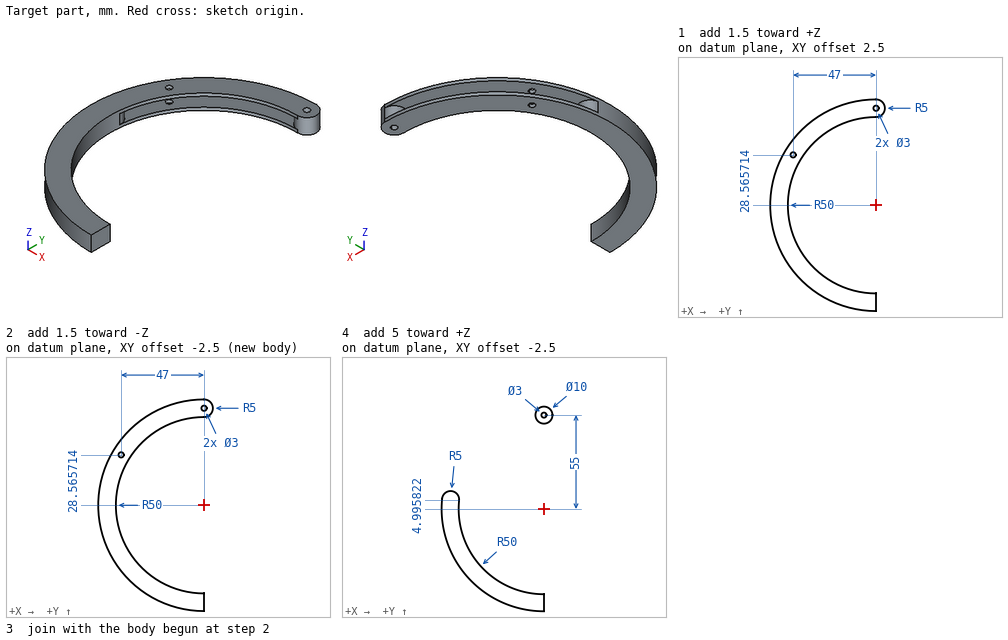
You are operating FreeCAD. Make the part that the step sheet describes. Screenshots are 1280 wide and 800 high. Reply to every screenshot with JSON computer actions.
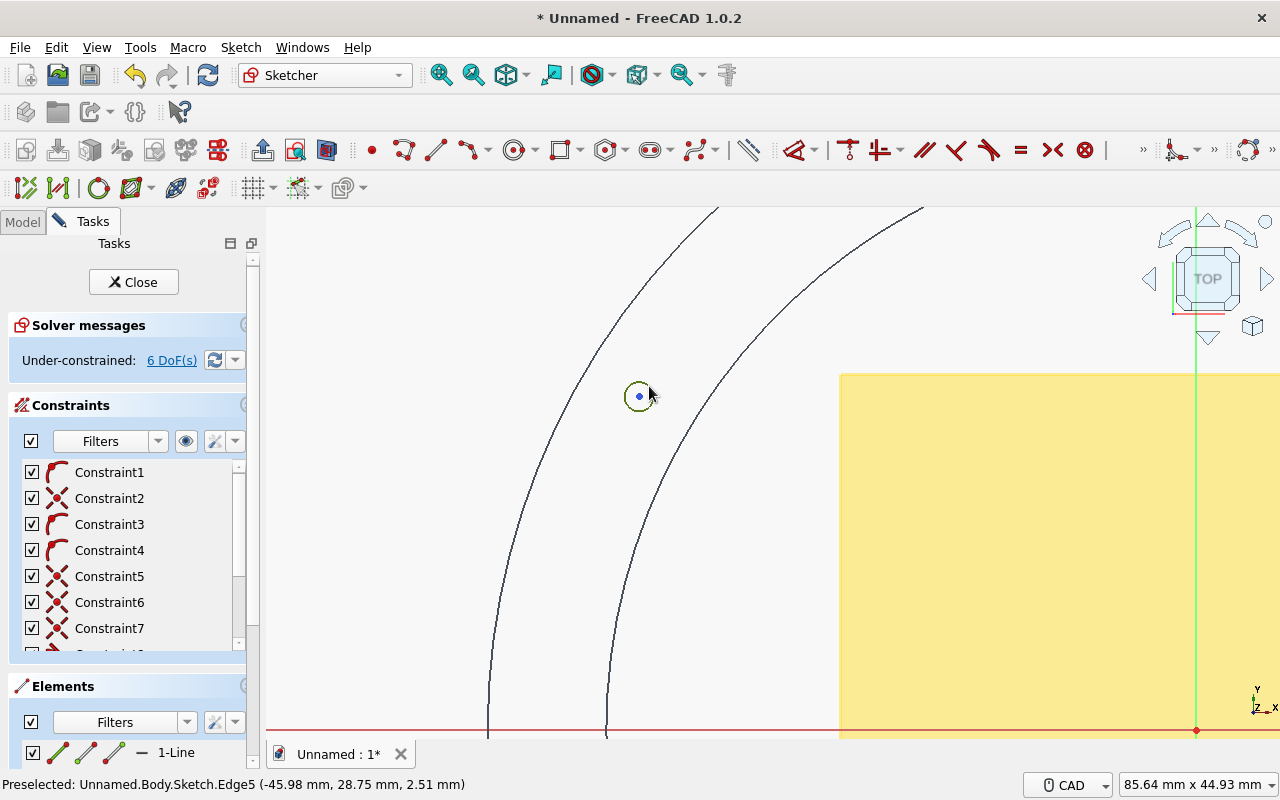
{"action": "scroll", "coordinate": [650, 389], "scroll_direction": "down", "scroll_amount": 7}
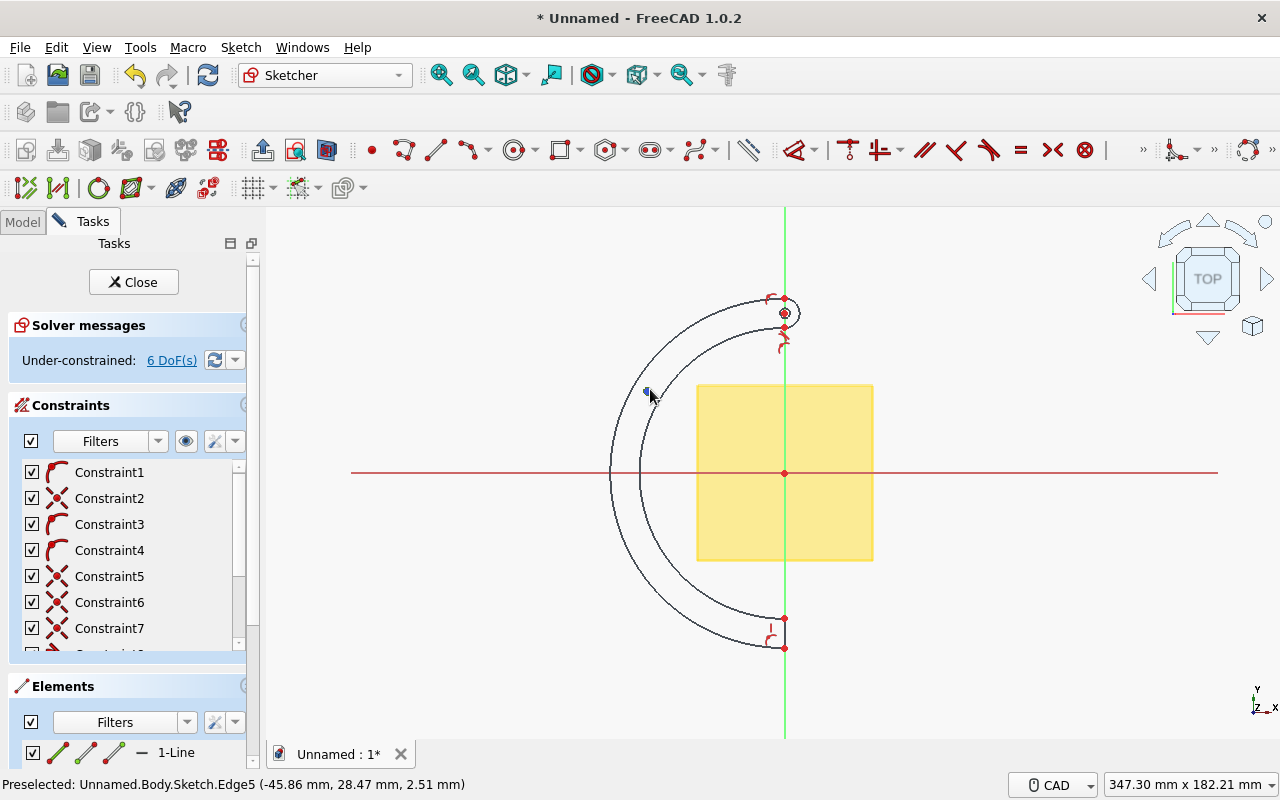
{"action": "scroll", "coordinate": [788, 310], "scroll_direction": "up", "scroll_amount": 7}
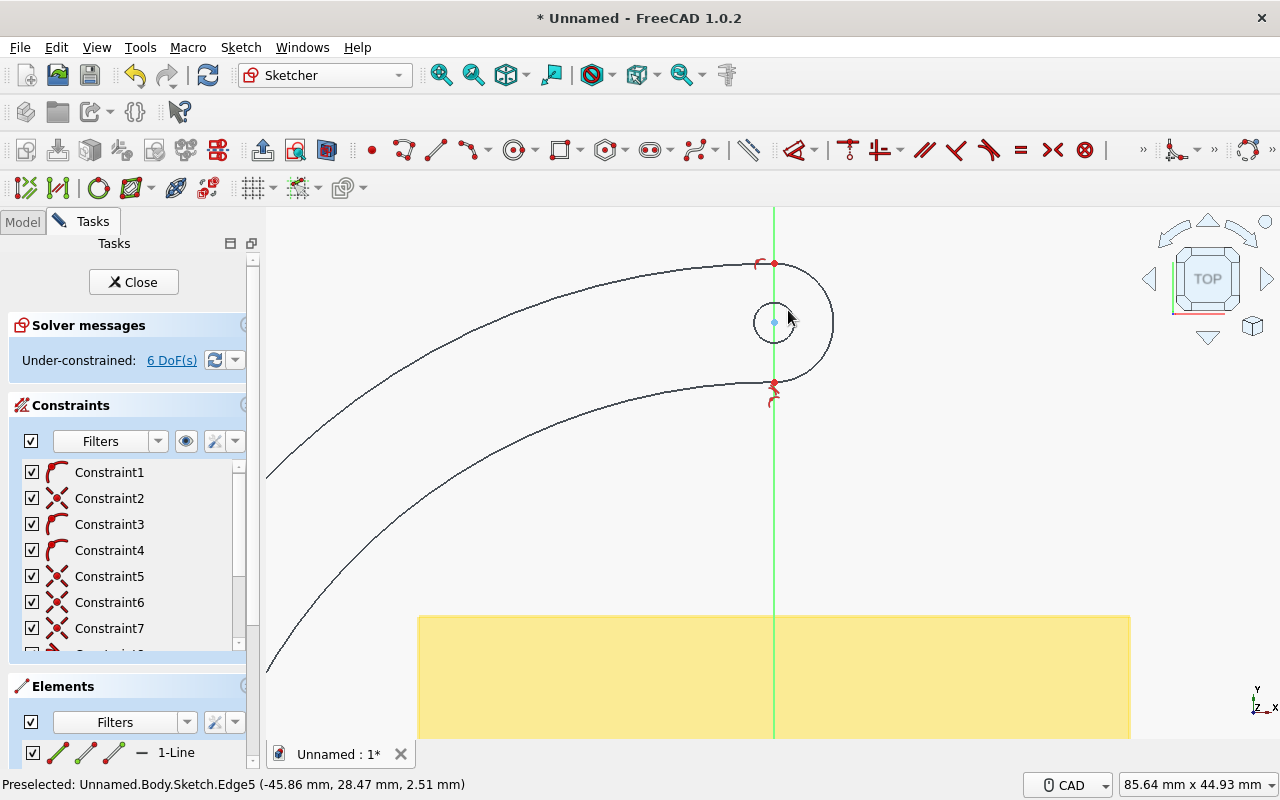
{"action": "left_click", "coordinate": [788, 309]}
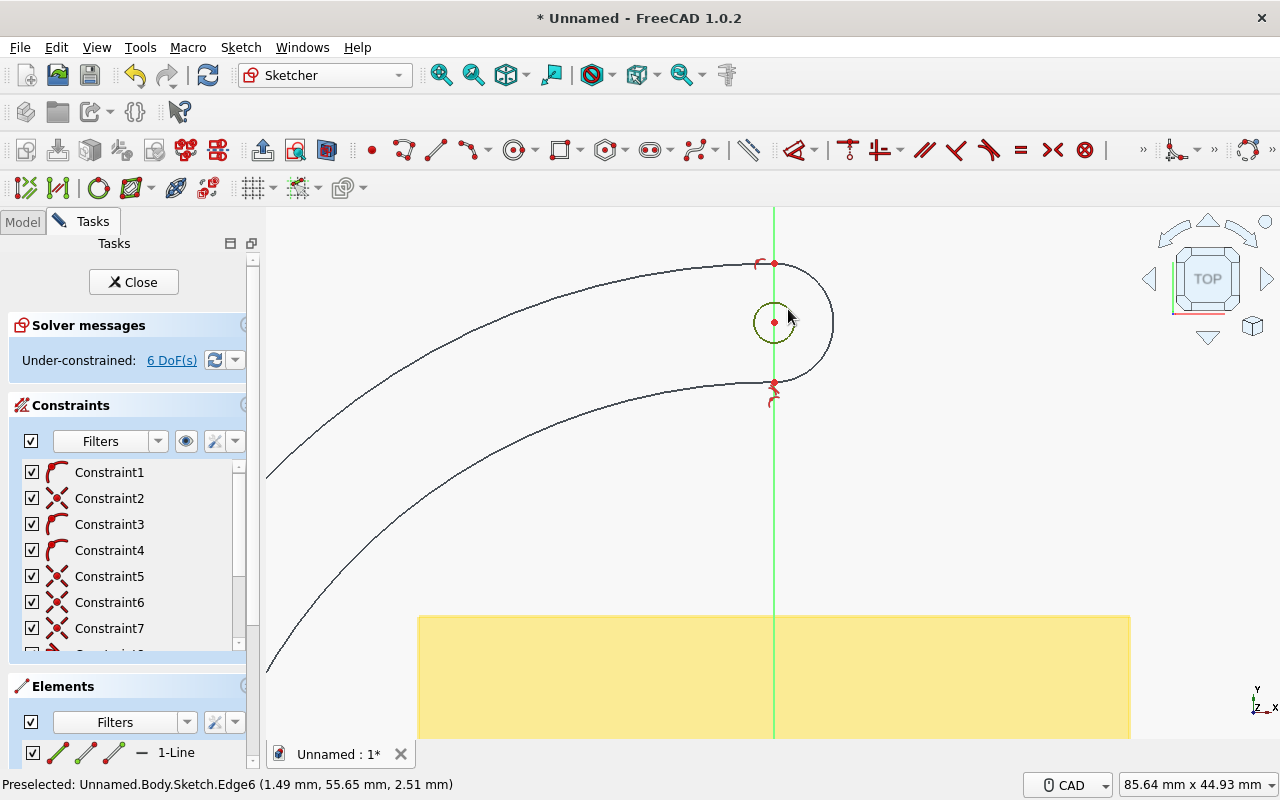
{"action": "left_click", "coordinate": [1022, 150]}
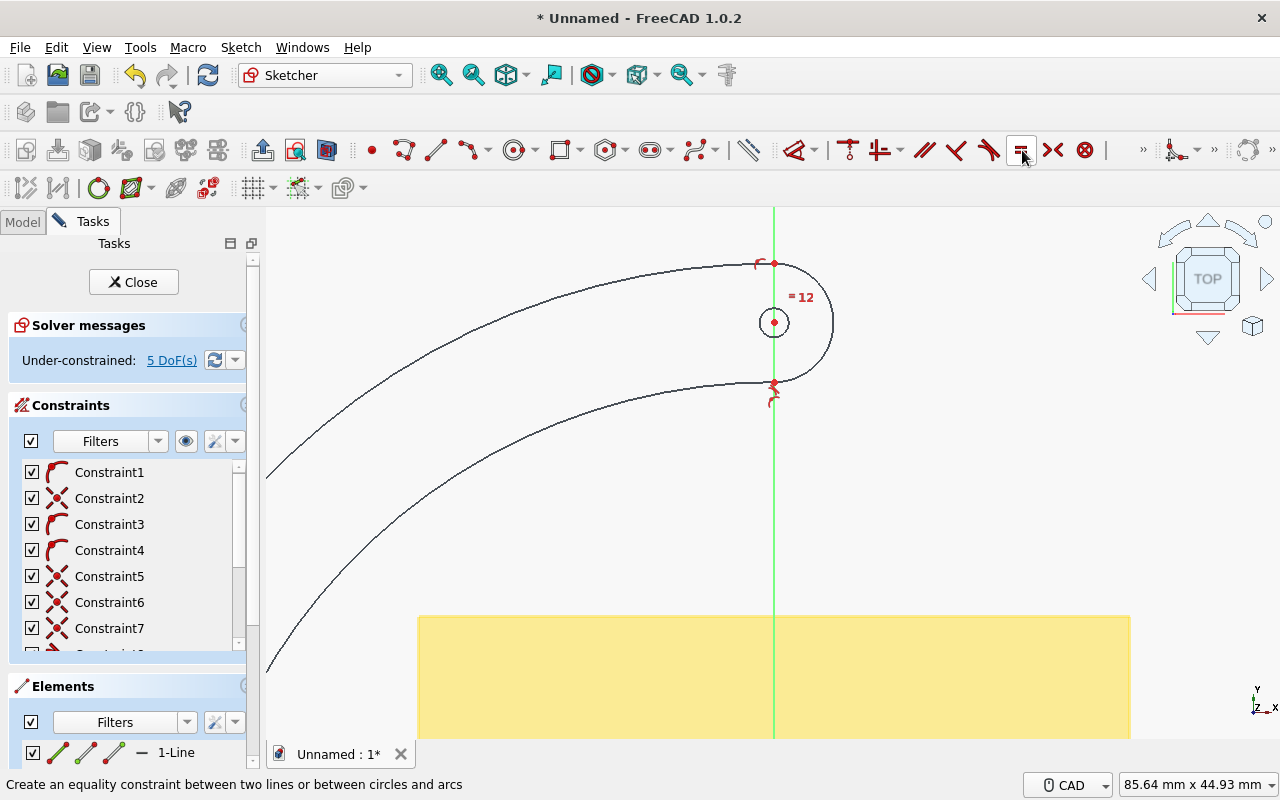
{"action": "left_click", "coordinate": [794, 150]}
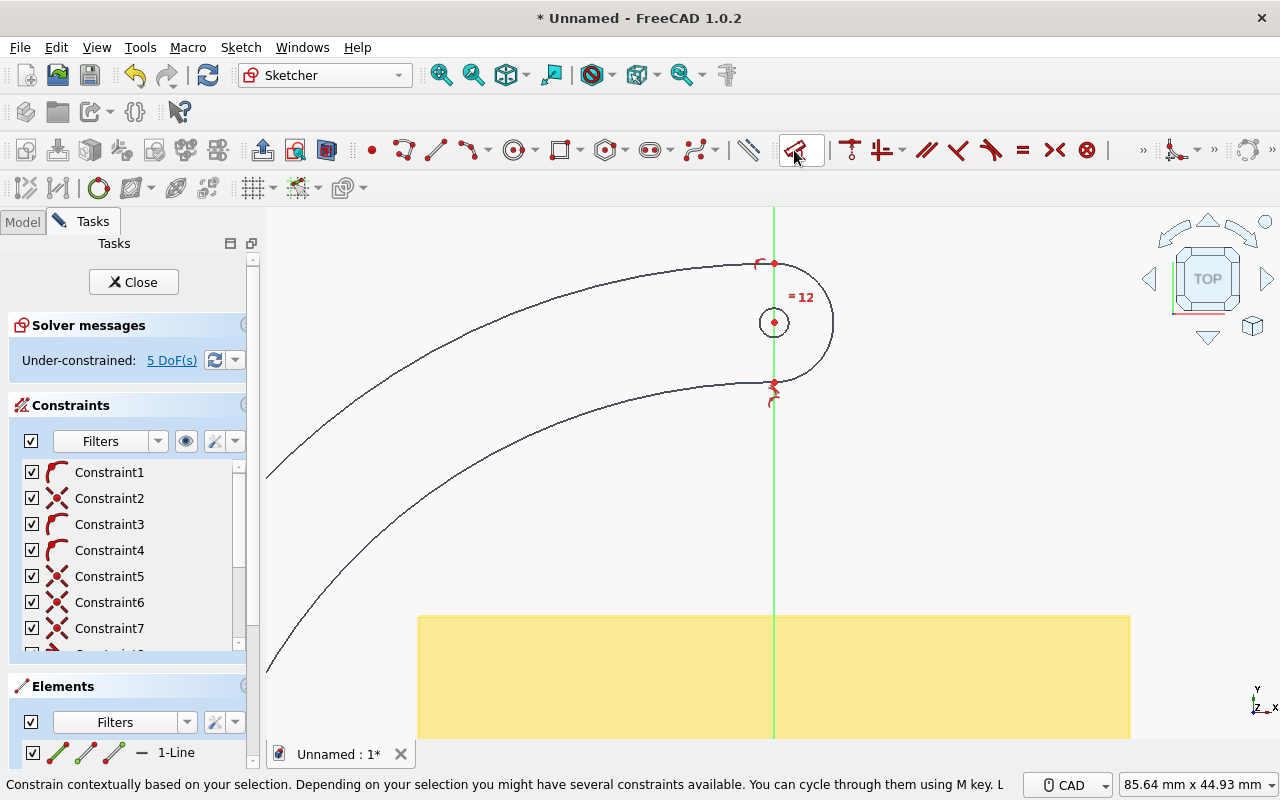
{"action": "scroll", "coordinate": [788, 310], "scroll_direction": "down", "scroll_amount": 7}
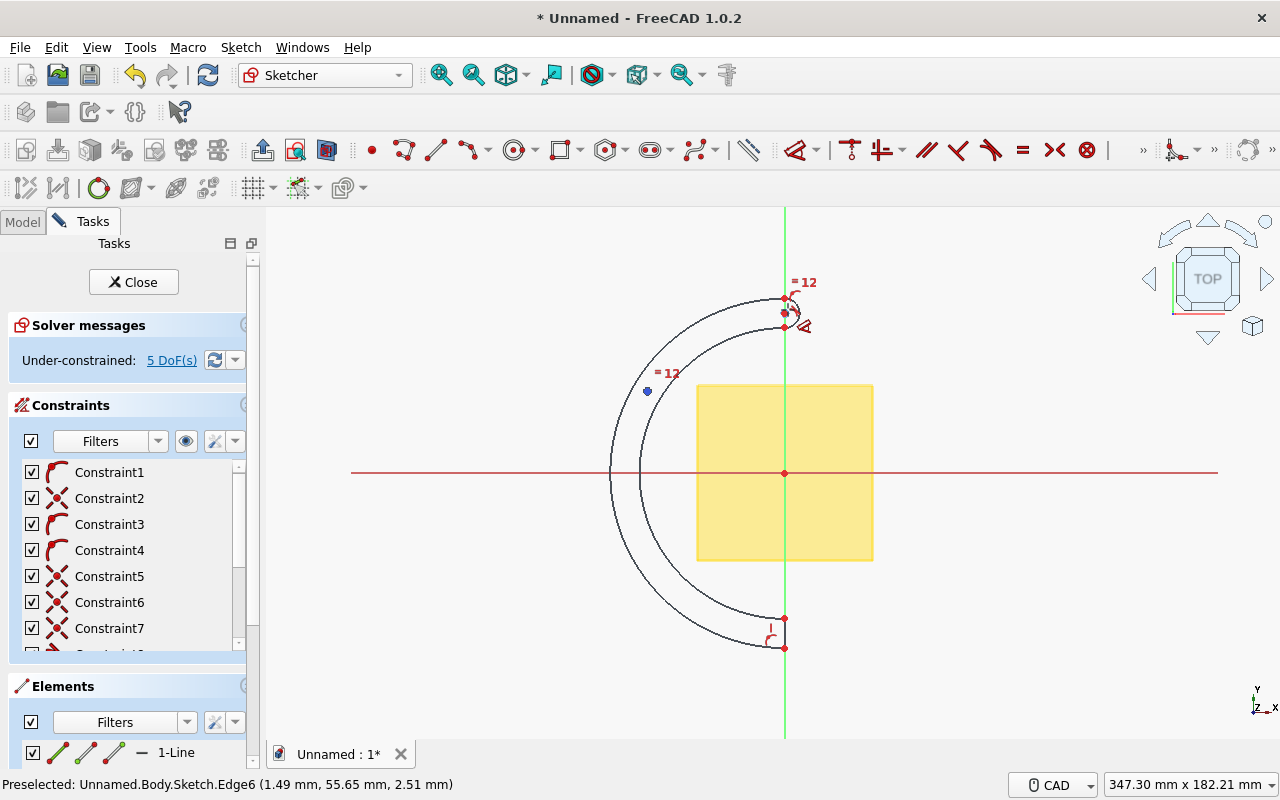
{"action": "left_click", "coordinate": [667, 388]}
{"action": "left_click", "coordinate": [889, 329]}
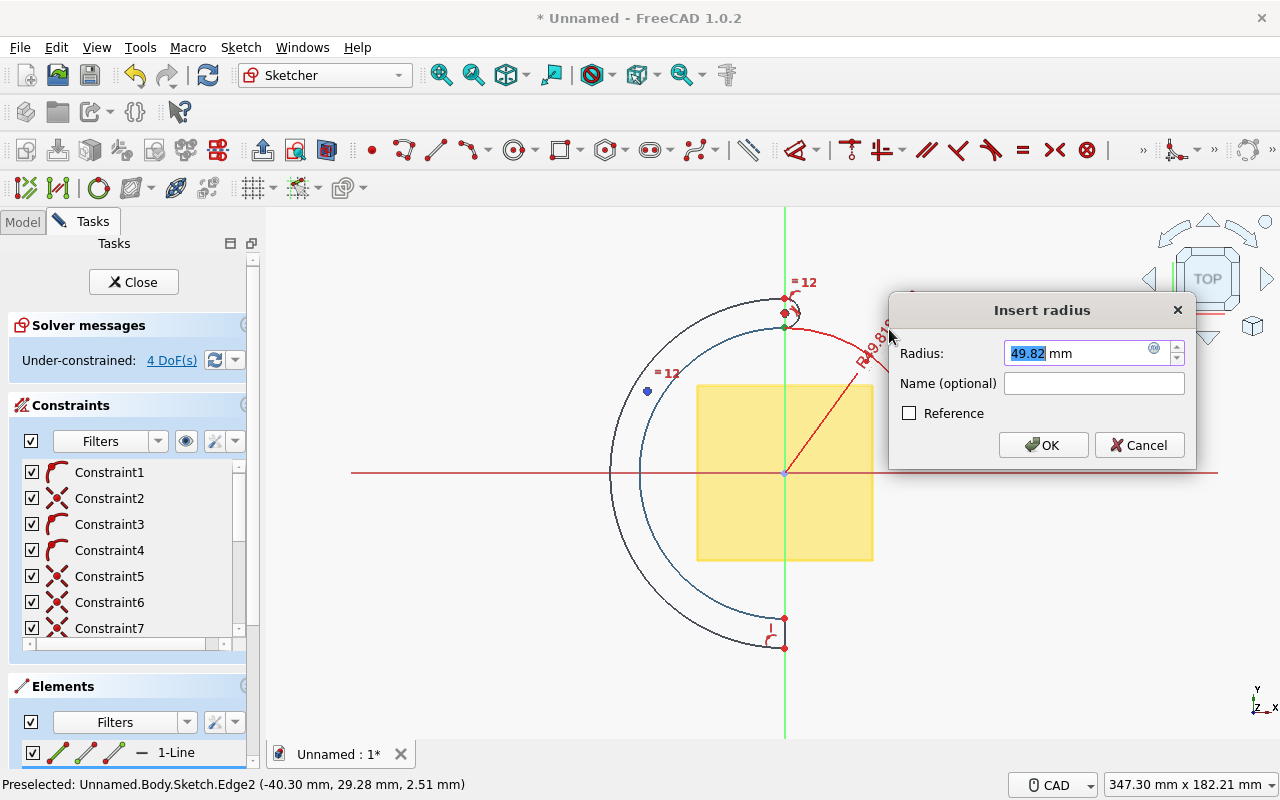
{"action": "type", "text": "50"}
{"action": "key", "text": "Return"}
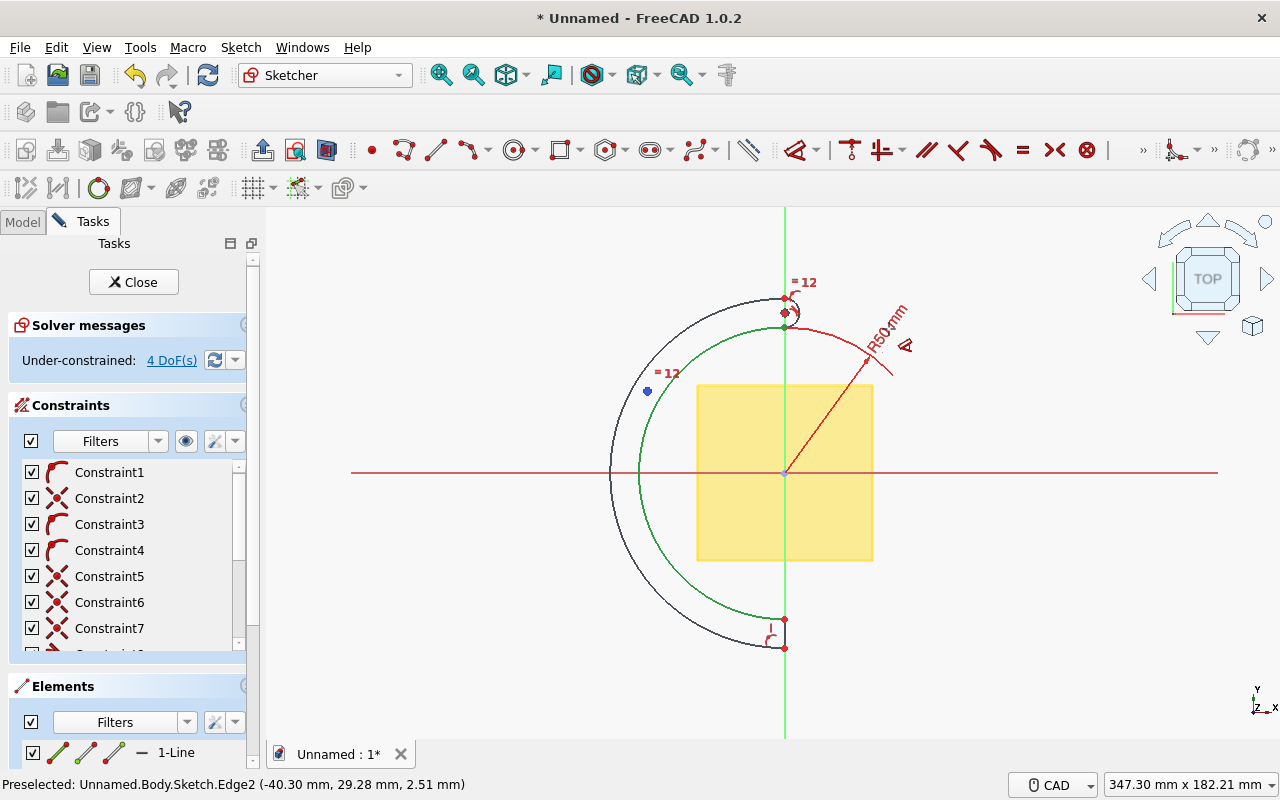
{"action": "scroll", "coordinate": [797, 321], "scroll_direction": "up", "scroll_amount": 6}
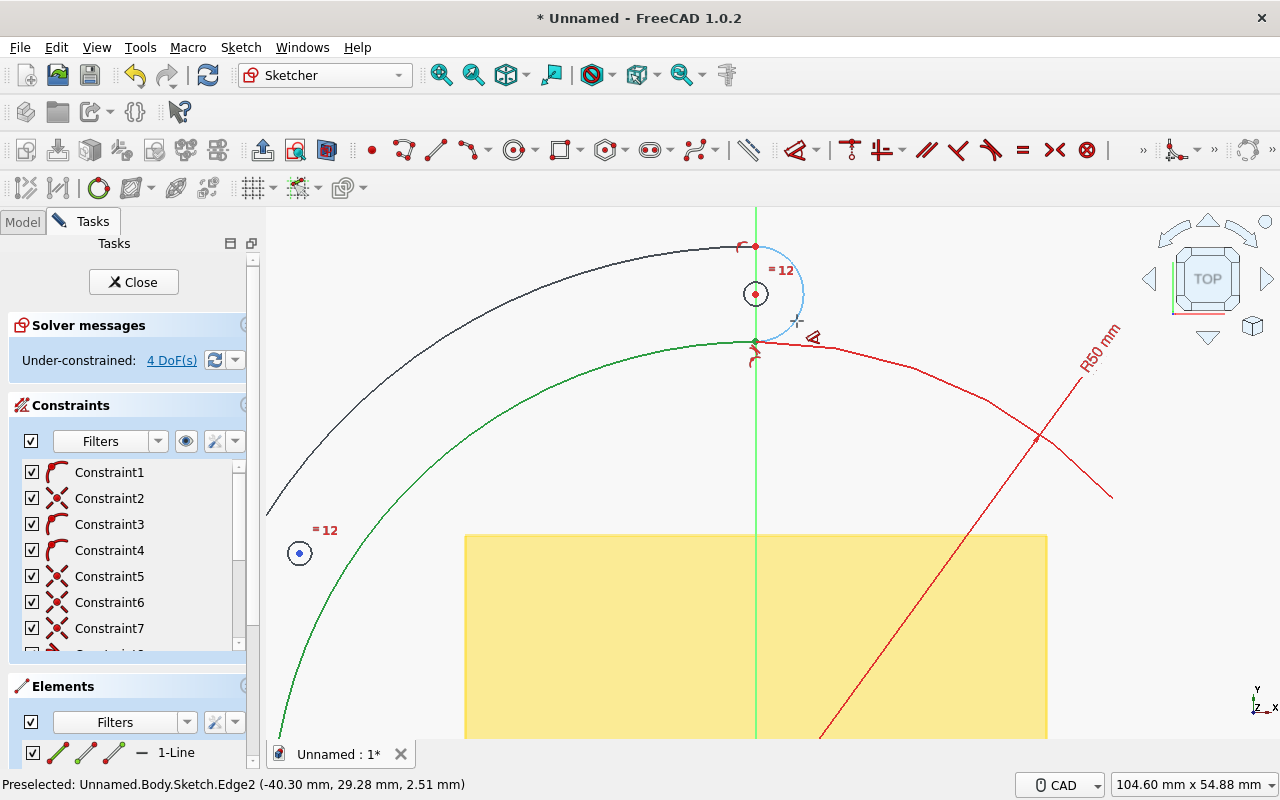
{"action": "left_click", "coordinate": [794, 322]}
{"action": "left_click", "coordinate": [820, 341]}